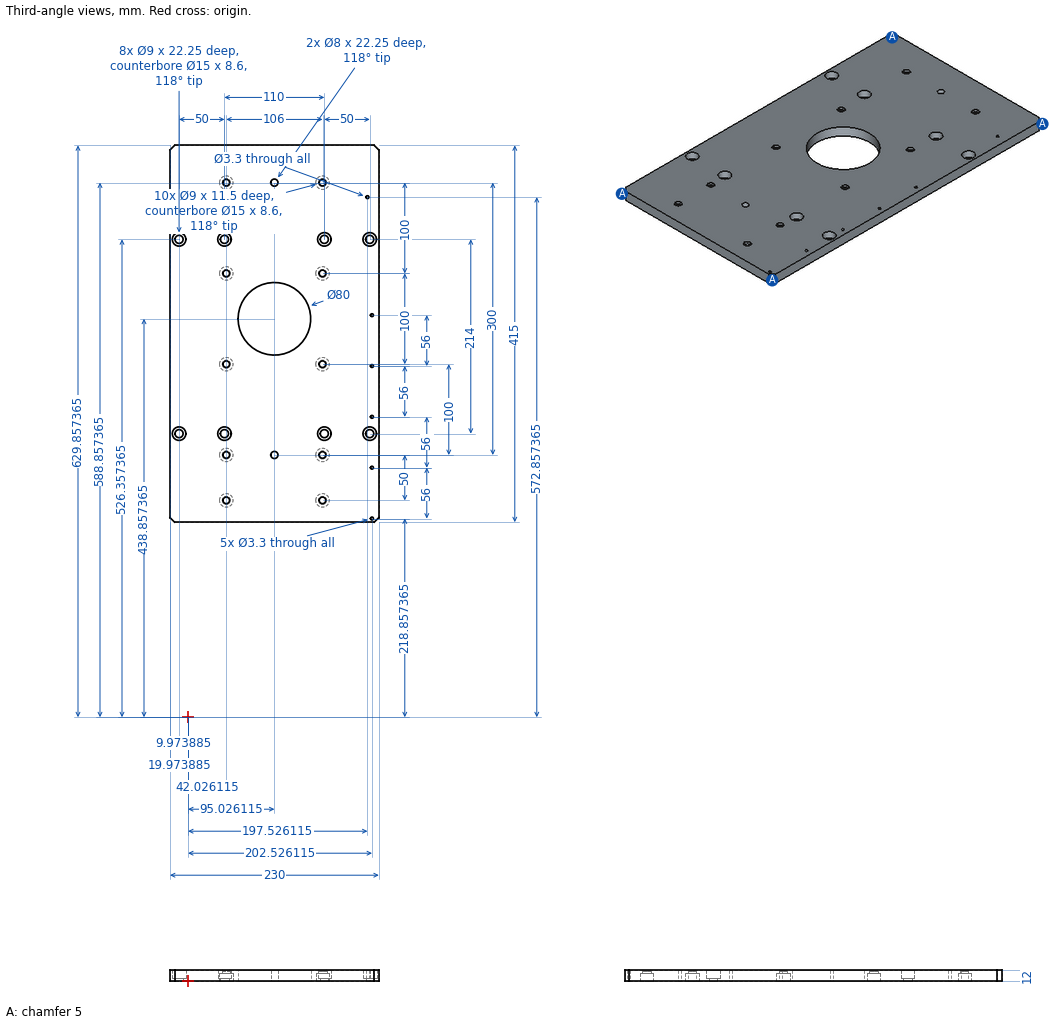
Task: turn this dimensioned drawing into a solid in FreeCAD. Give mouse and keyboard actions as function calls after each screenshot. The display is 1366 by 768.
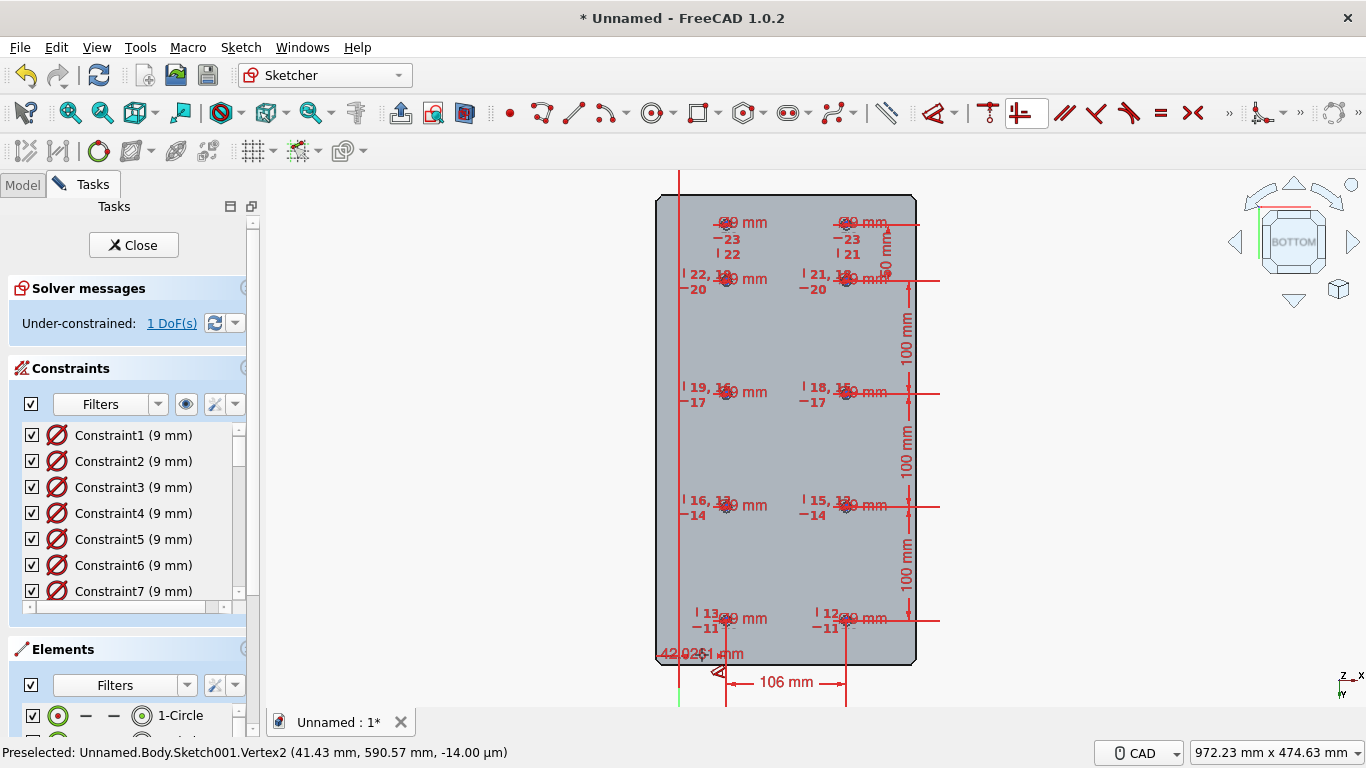
click(846, 621)
click(645, 409)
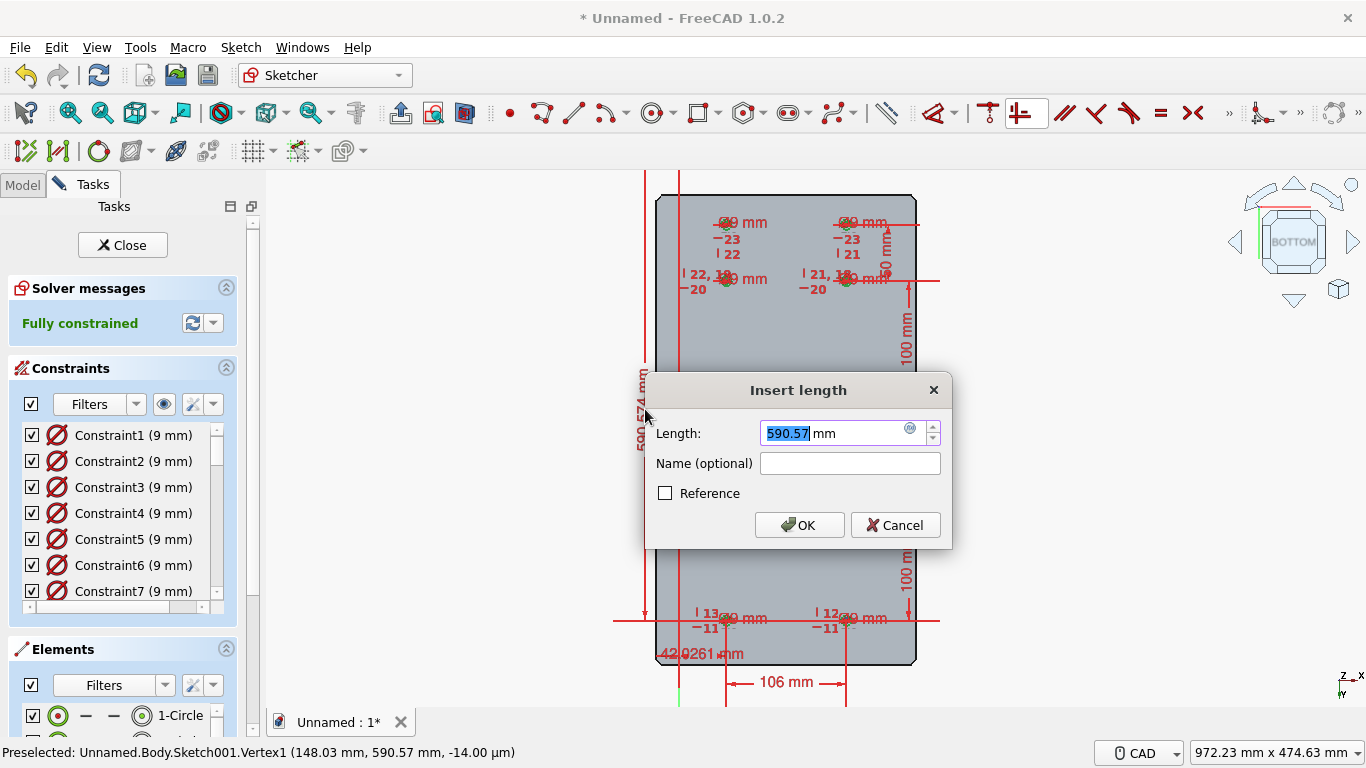
text(588.857365)
key(Return)
key(Escape)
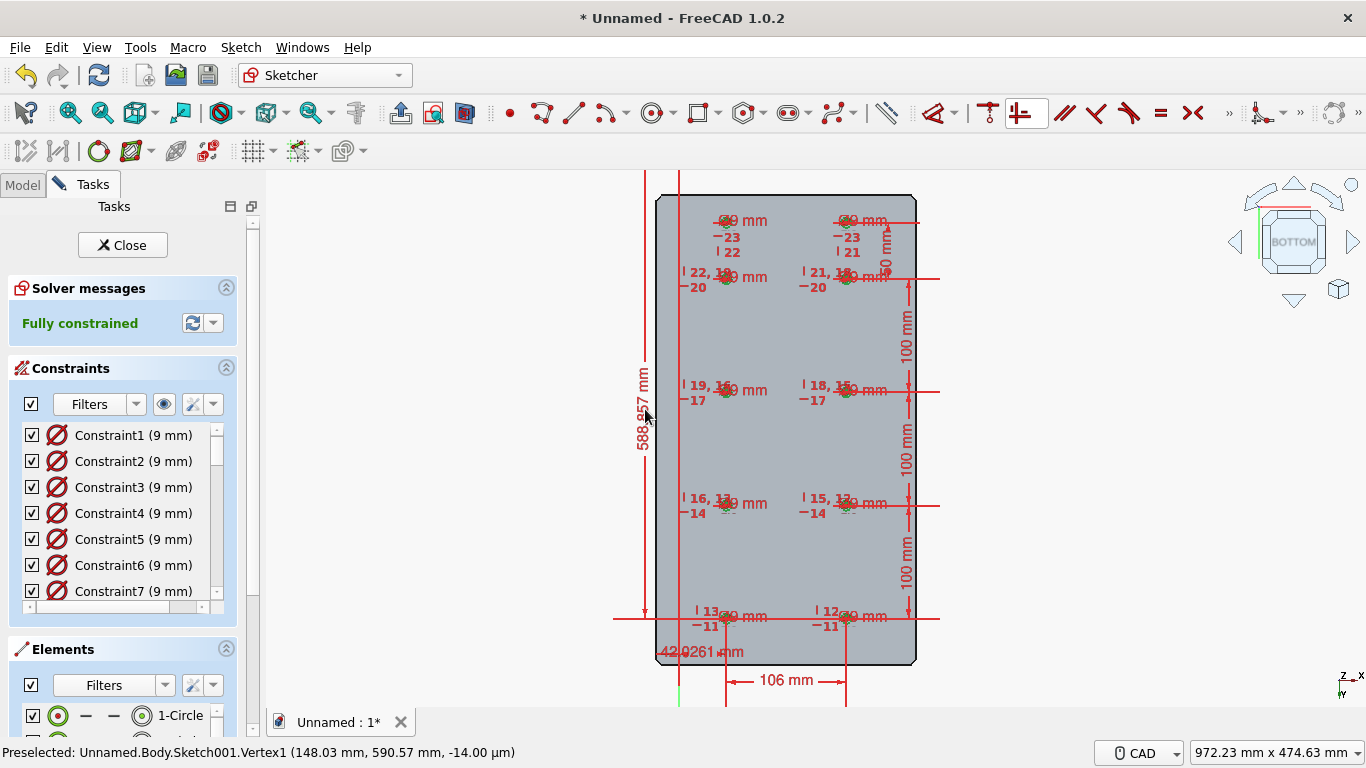
click(123, 245)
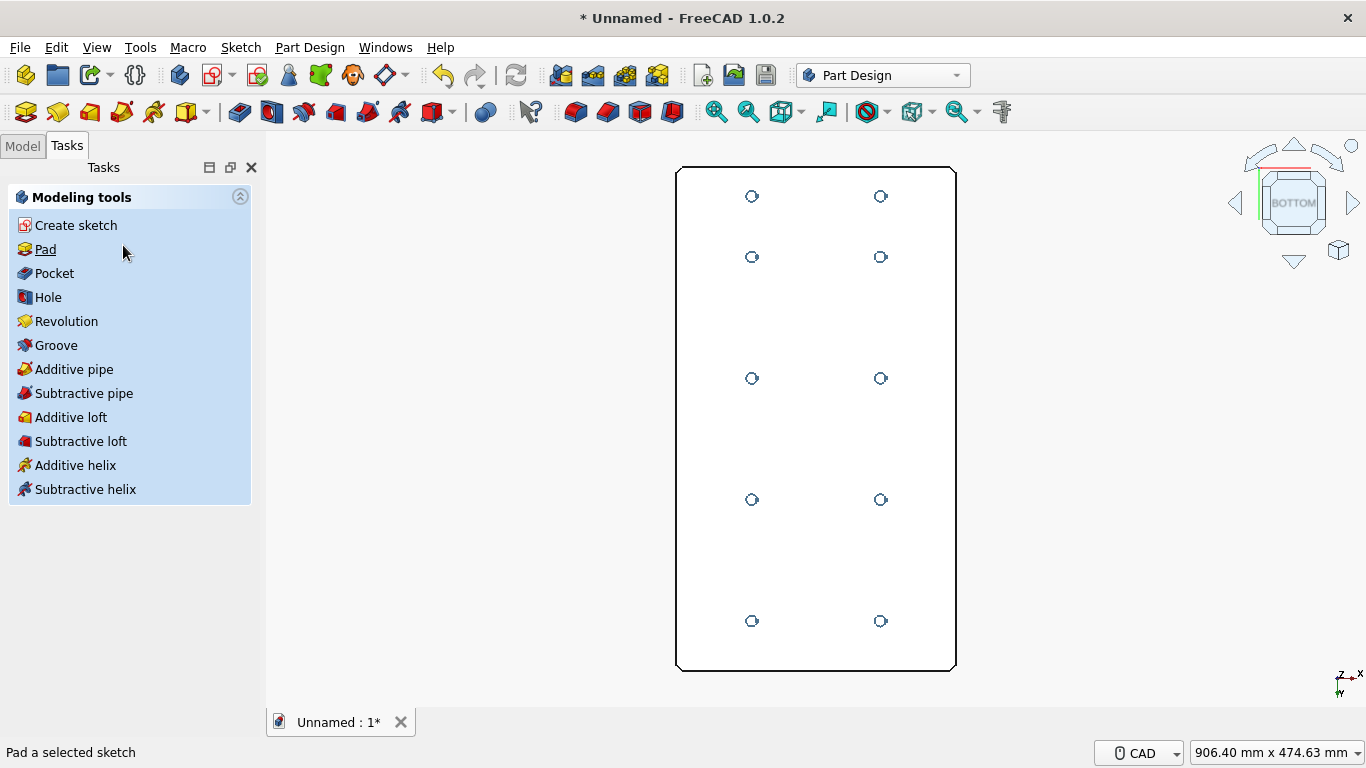
click(272, 112)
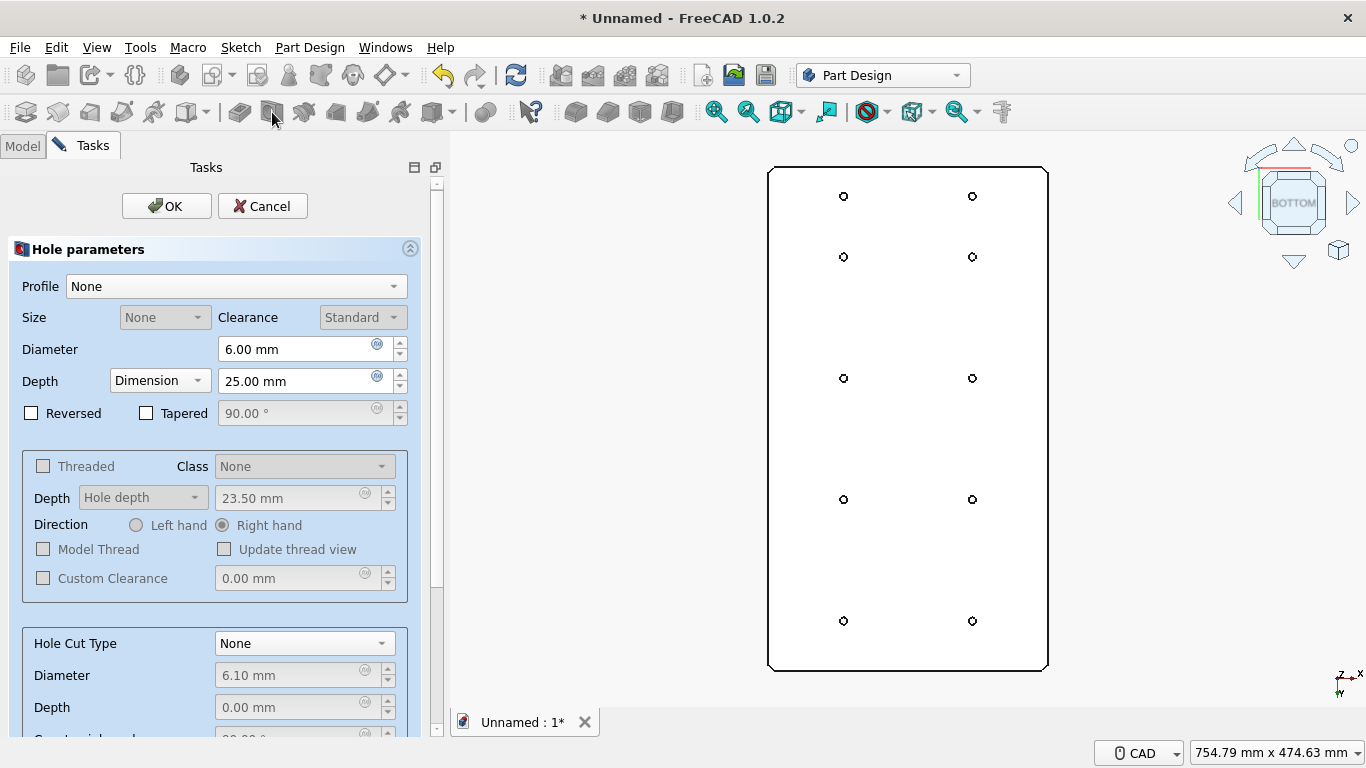
triple_click(305, 349)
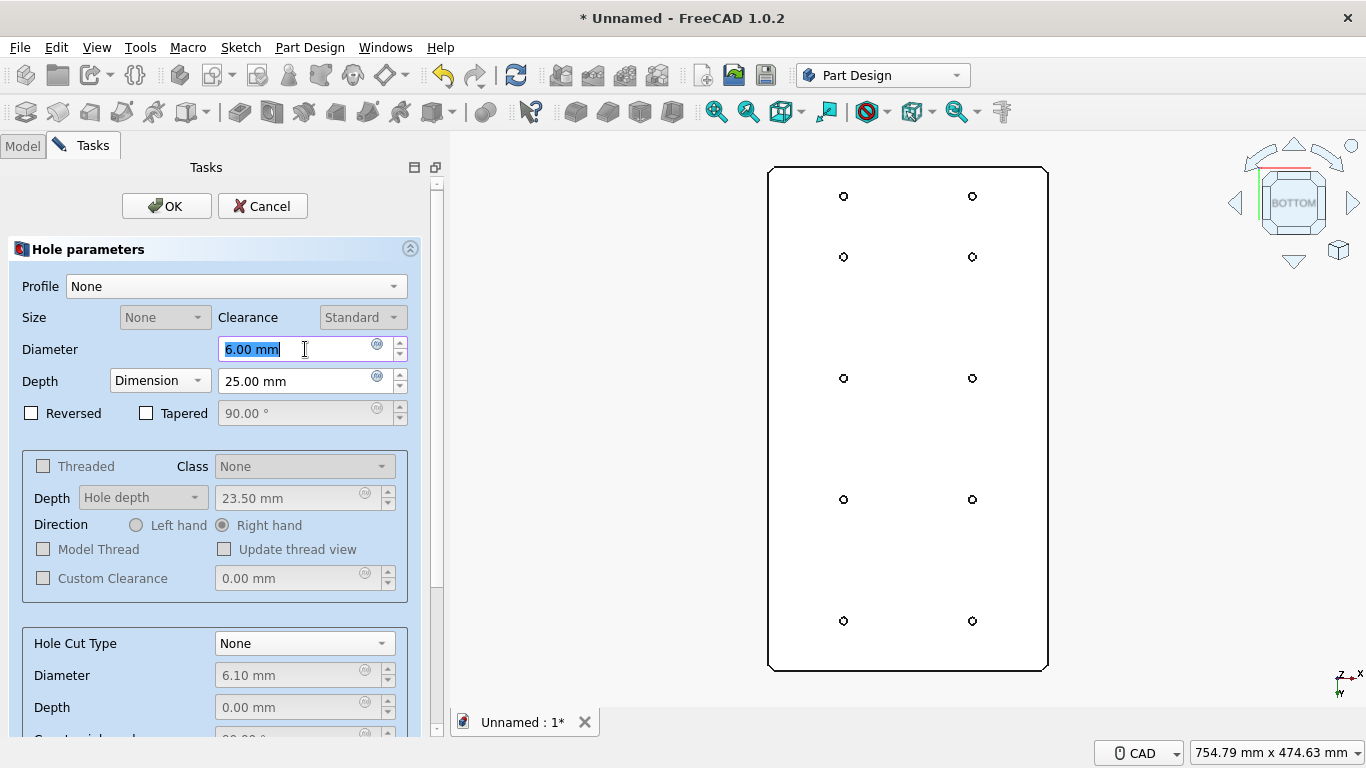
text(9)
key(Tab)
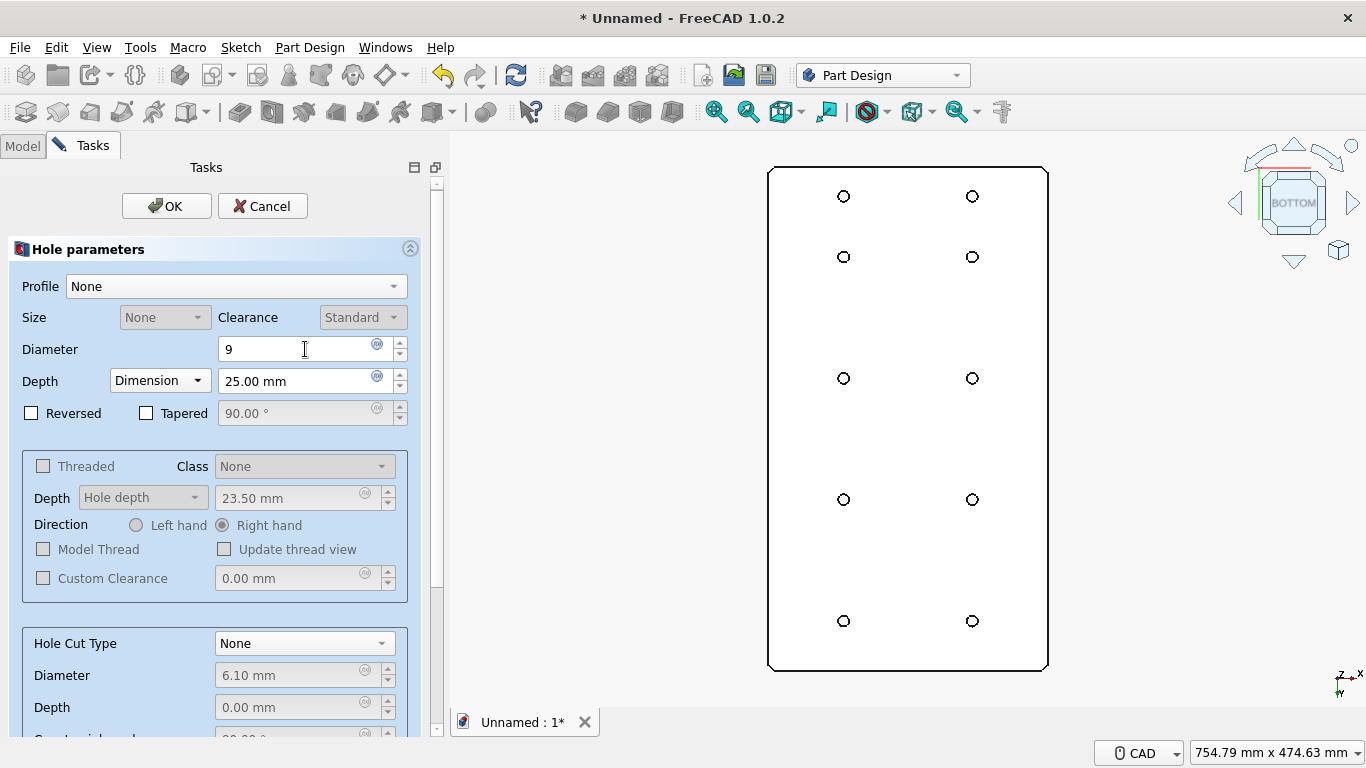
triple_click(305, 381)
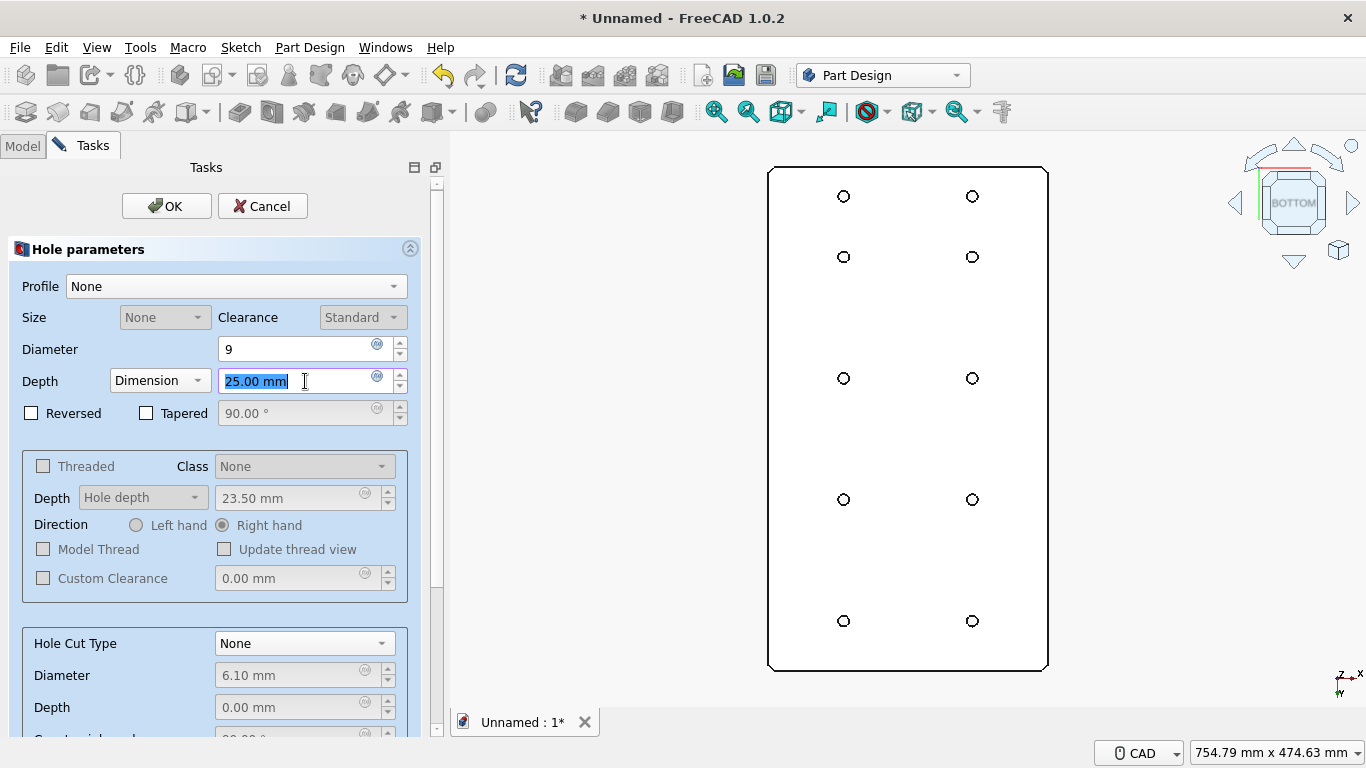
text(11.5)
key(Tab)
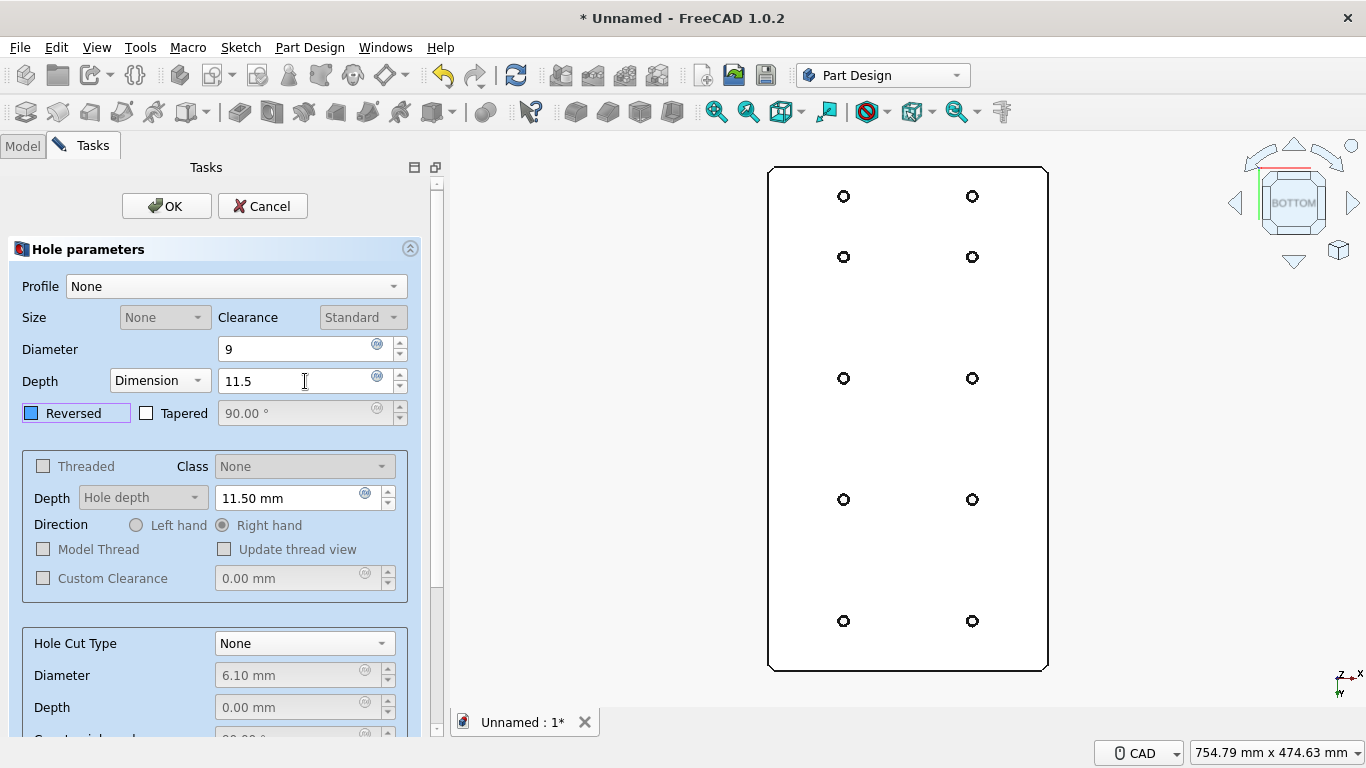
click(306, 644)